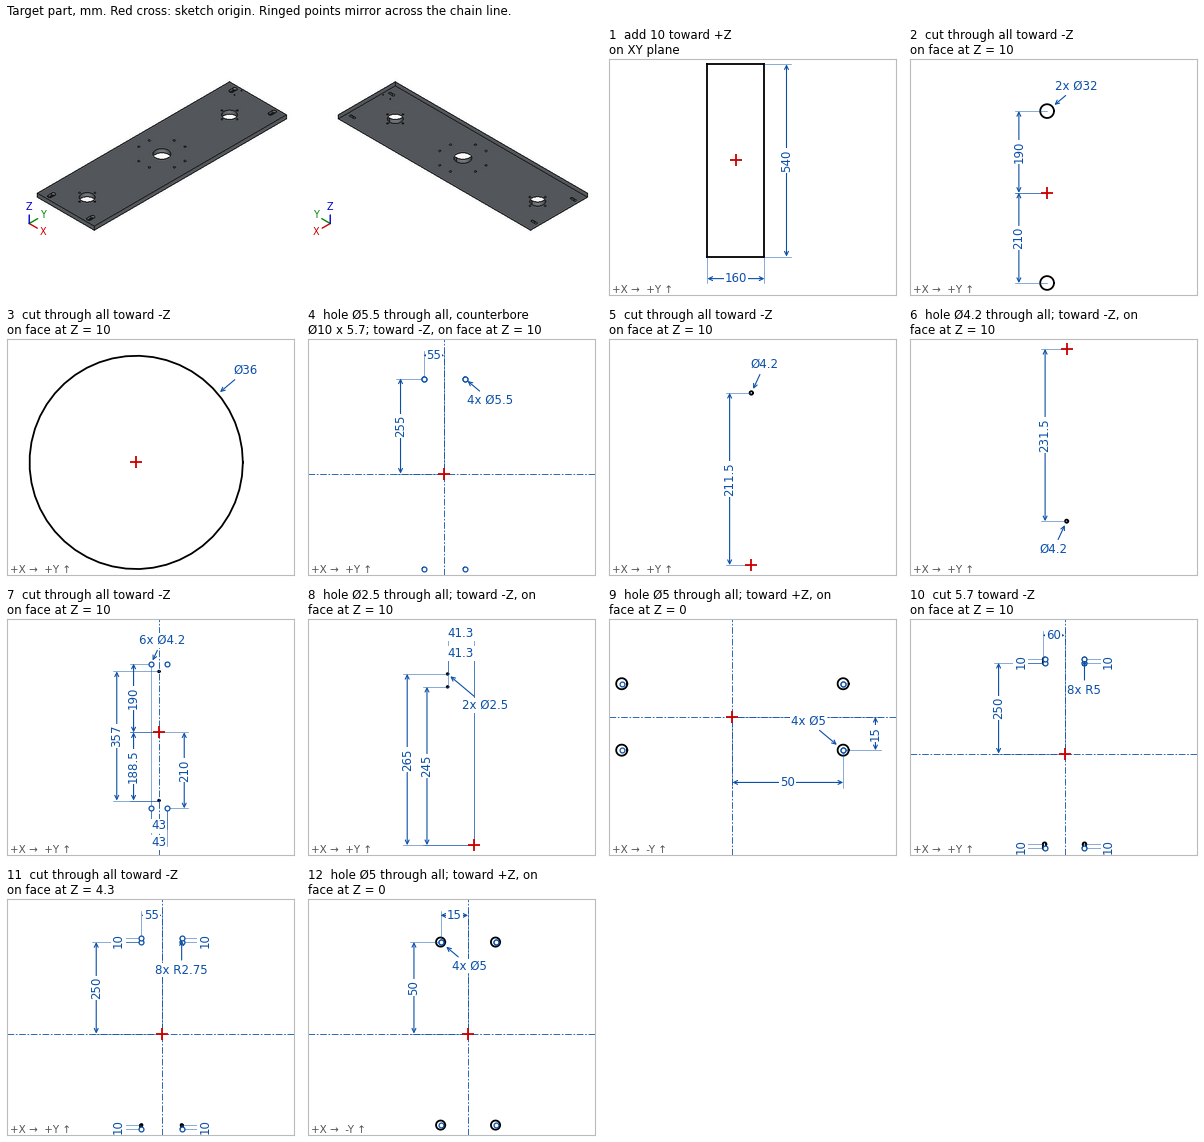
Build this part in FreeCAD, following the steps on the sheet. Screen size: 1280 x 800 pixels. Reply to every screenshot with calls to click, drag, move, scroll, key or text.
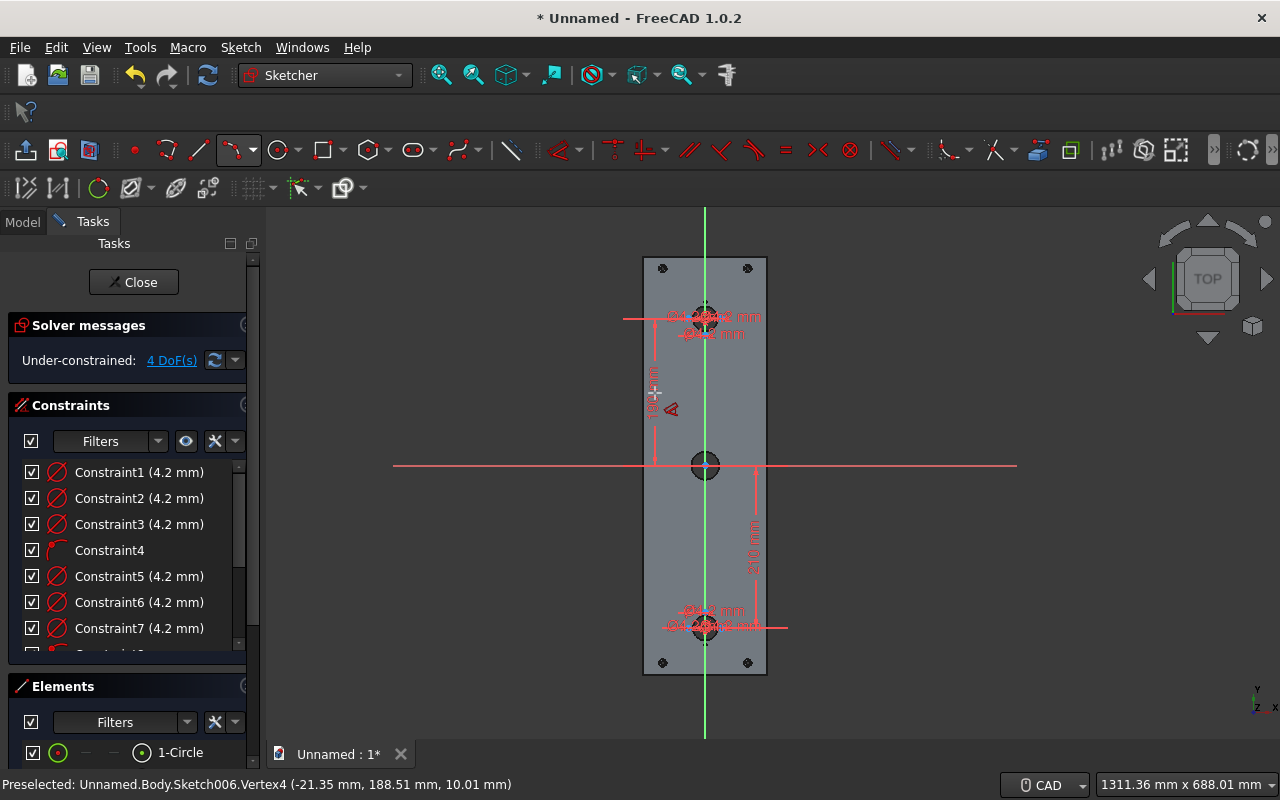
click(722, 628)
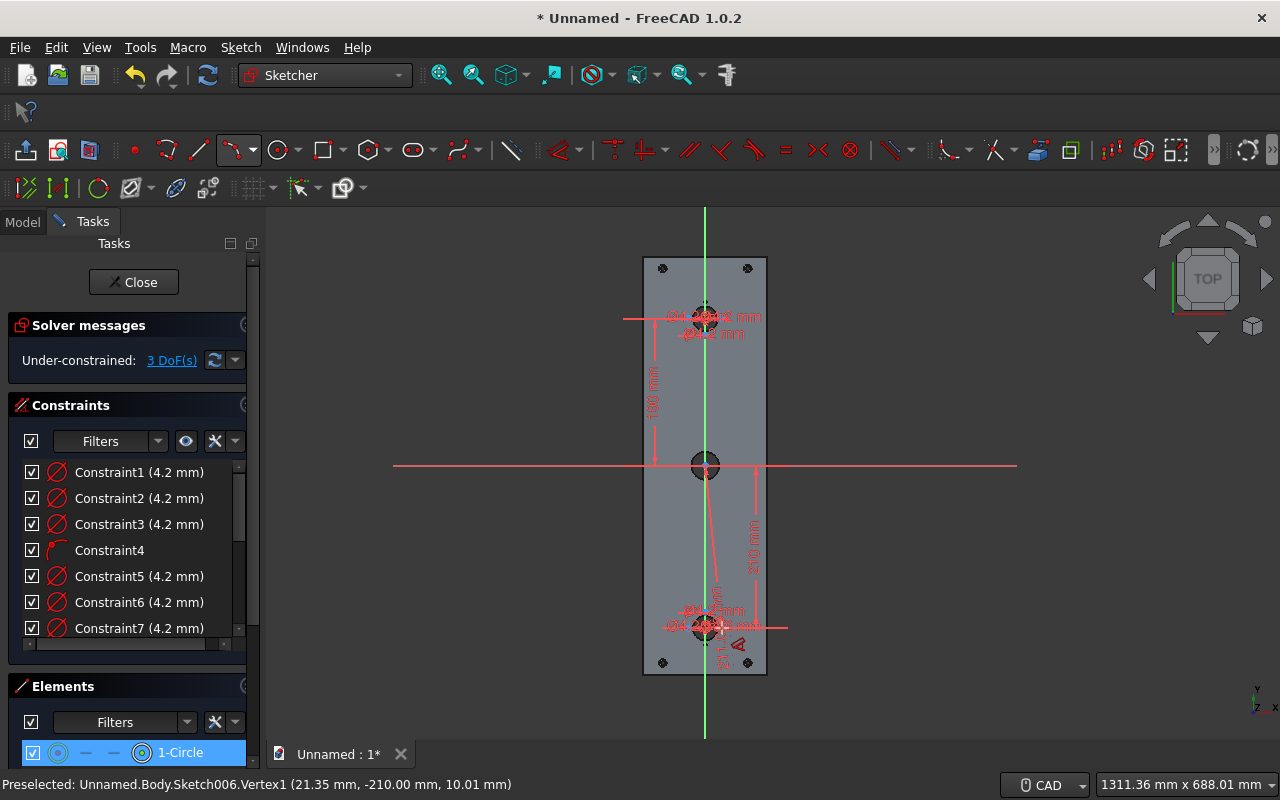
click(689, 628)
click(698, 662)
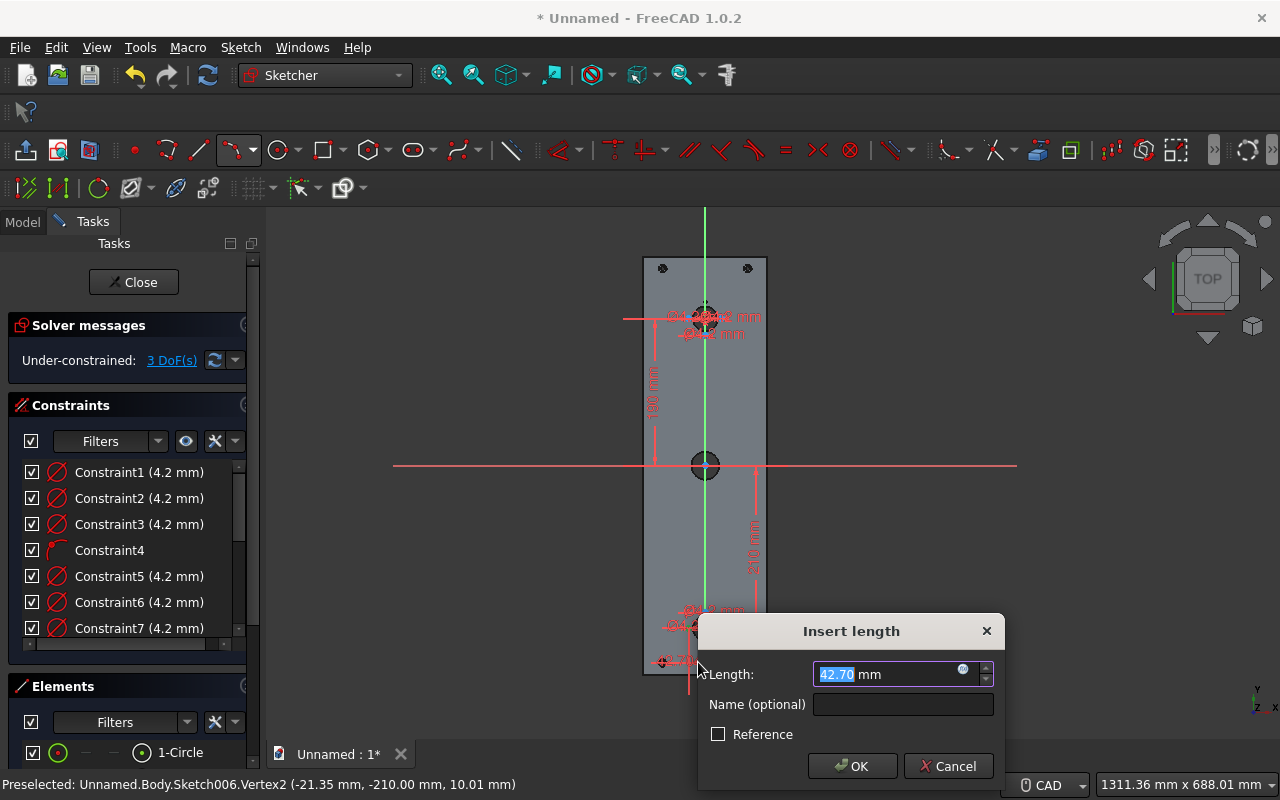
text(43)
key(Return)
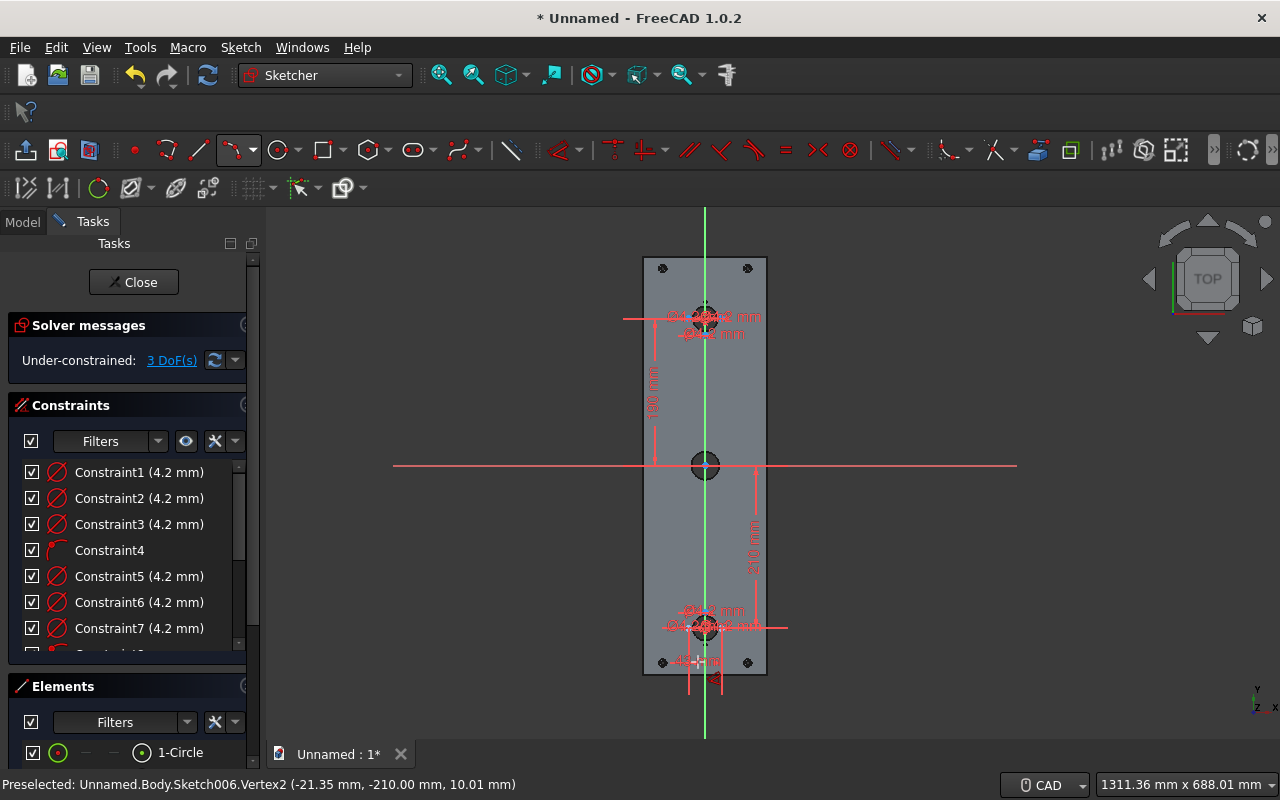
click(722, 628)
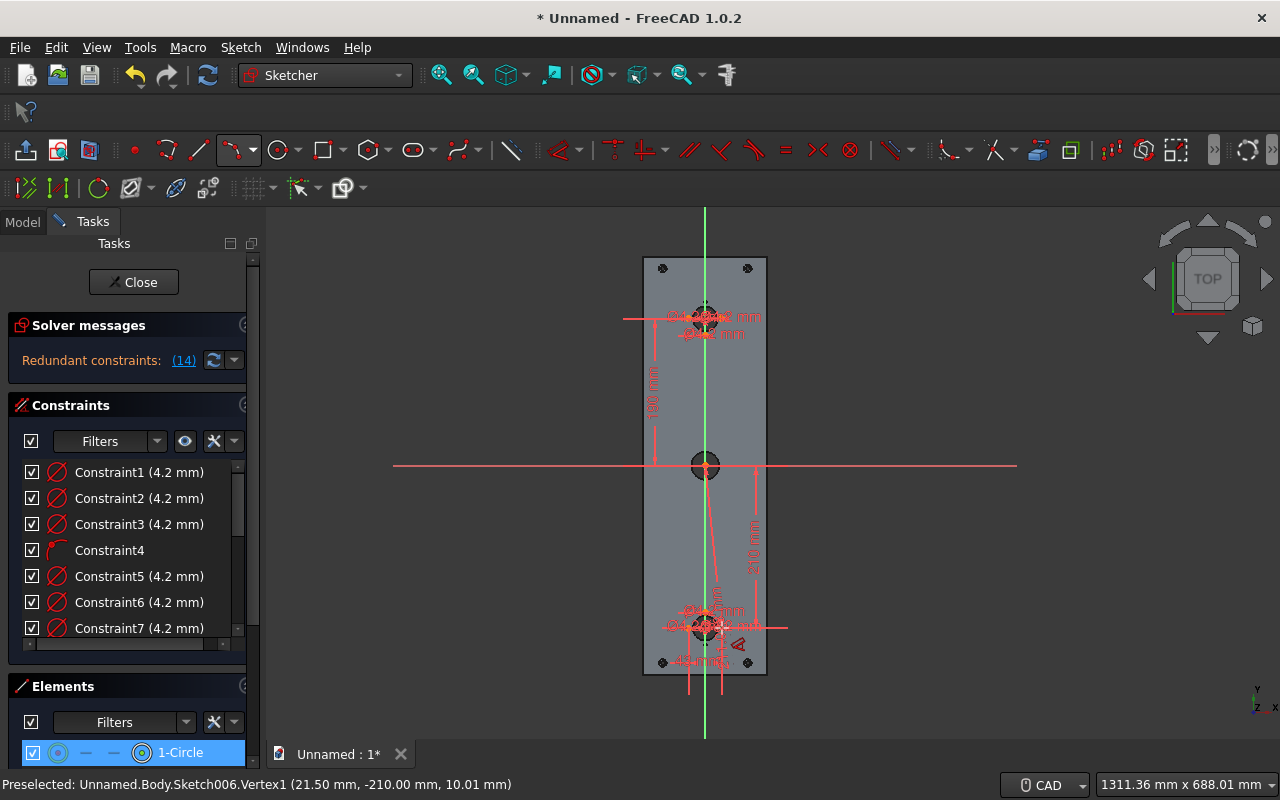
click(689, 319)
click(698, 285)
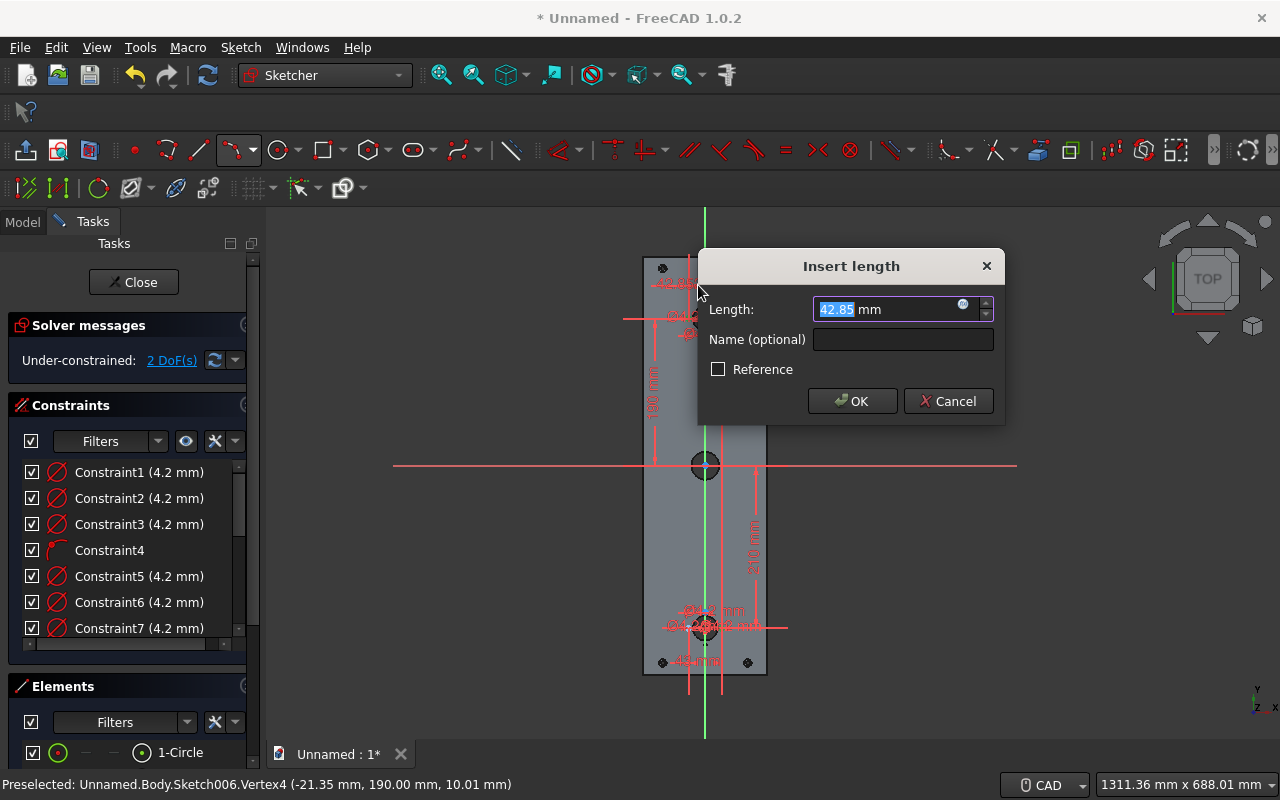
text(43)
key(Return)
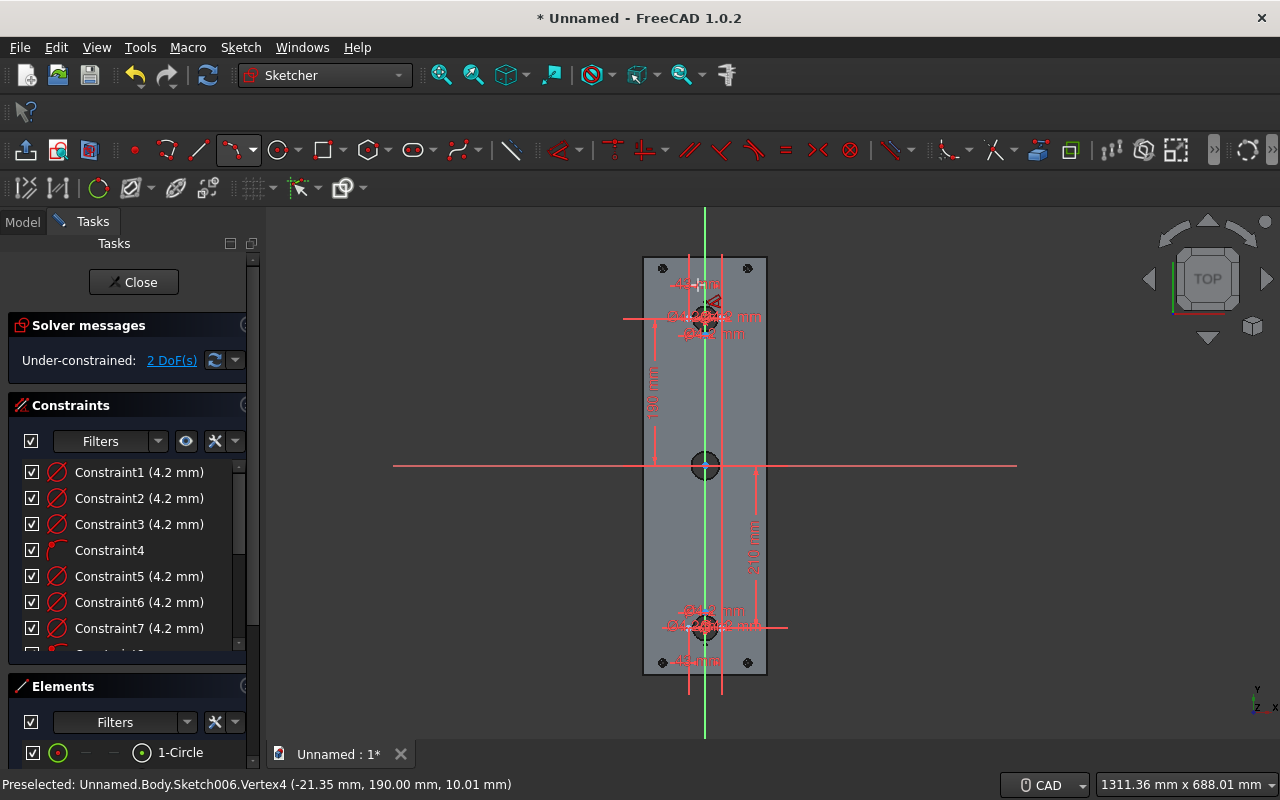
click(705, 613)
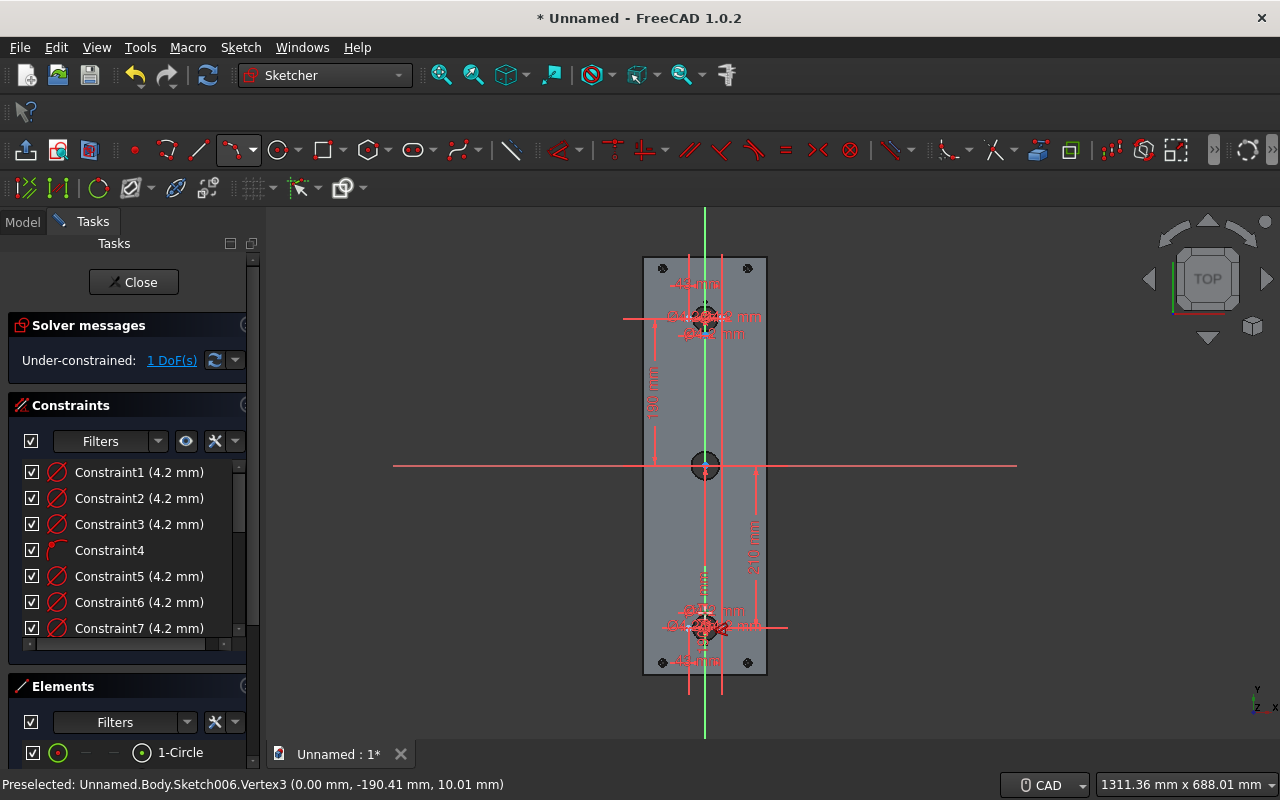
click(705, 336)
click(739, 411)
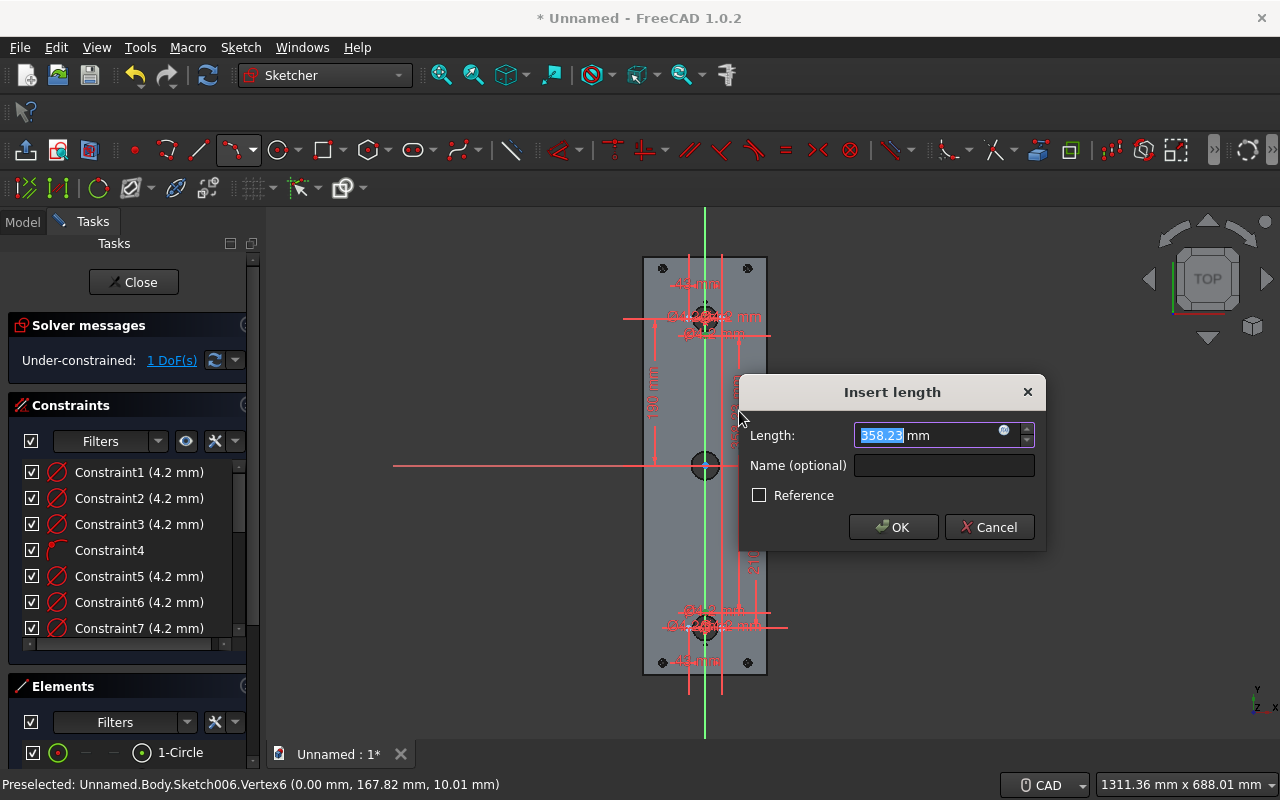
text(357)
key(Return)